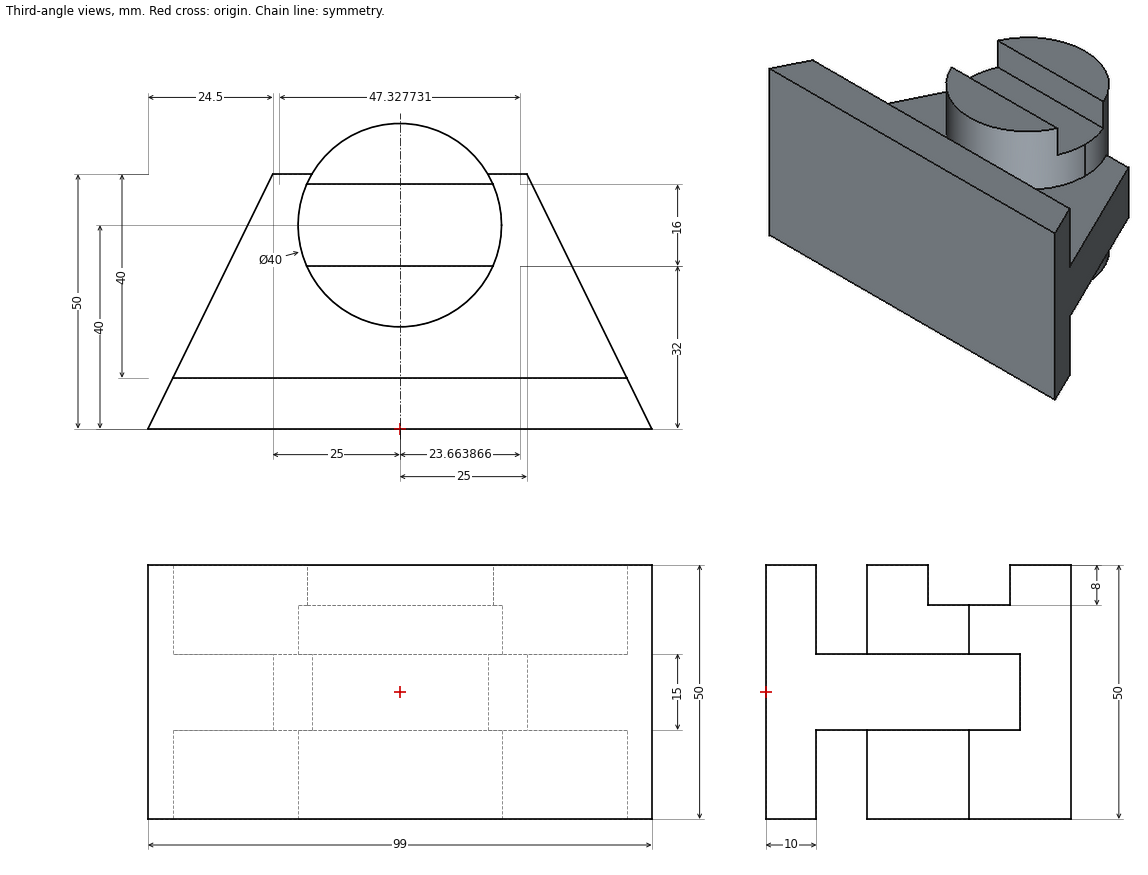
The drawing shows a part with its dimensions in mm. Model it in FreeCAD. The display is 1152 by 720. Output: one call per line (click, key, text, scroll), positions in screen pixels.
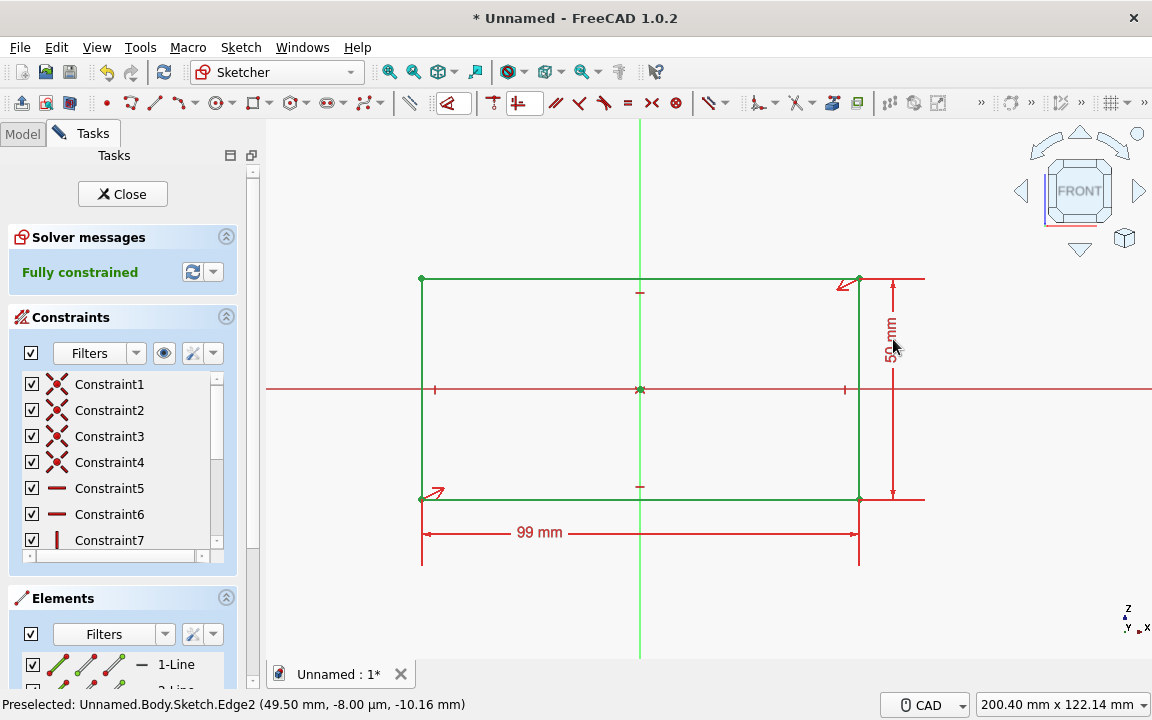
click(123, 194)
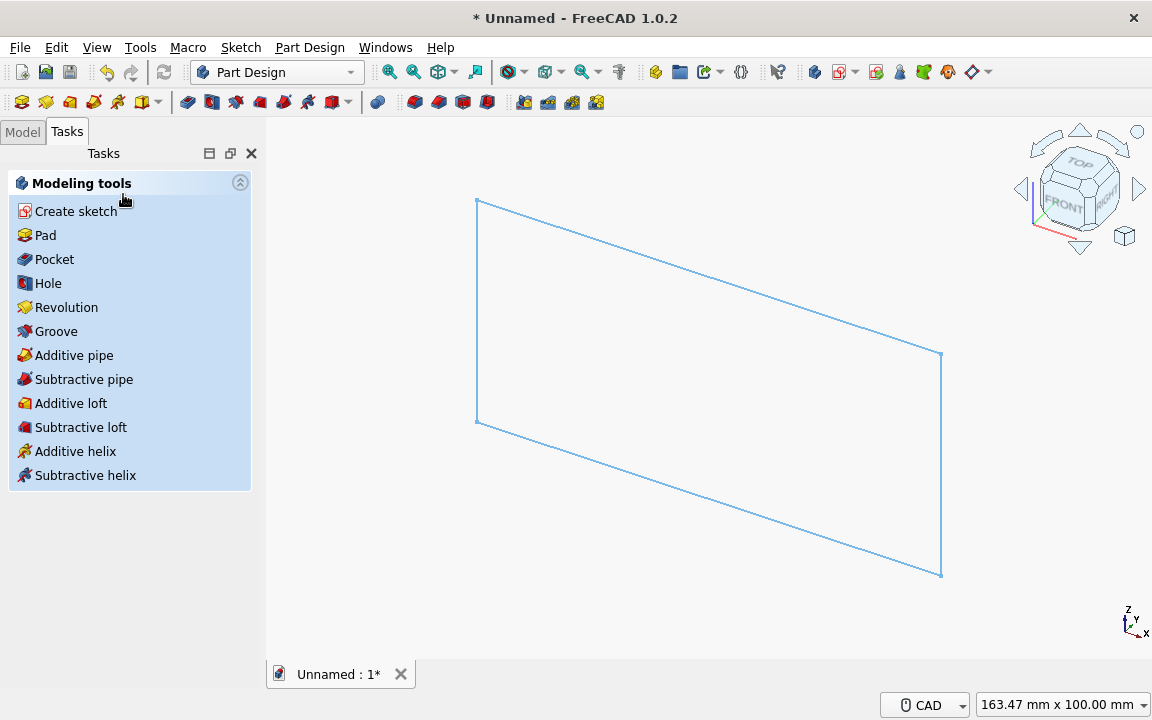
click(22, 102)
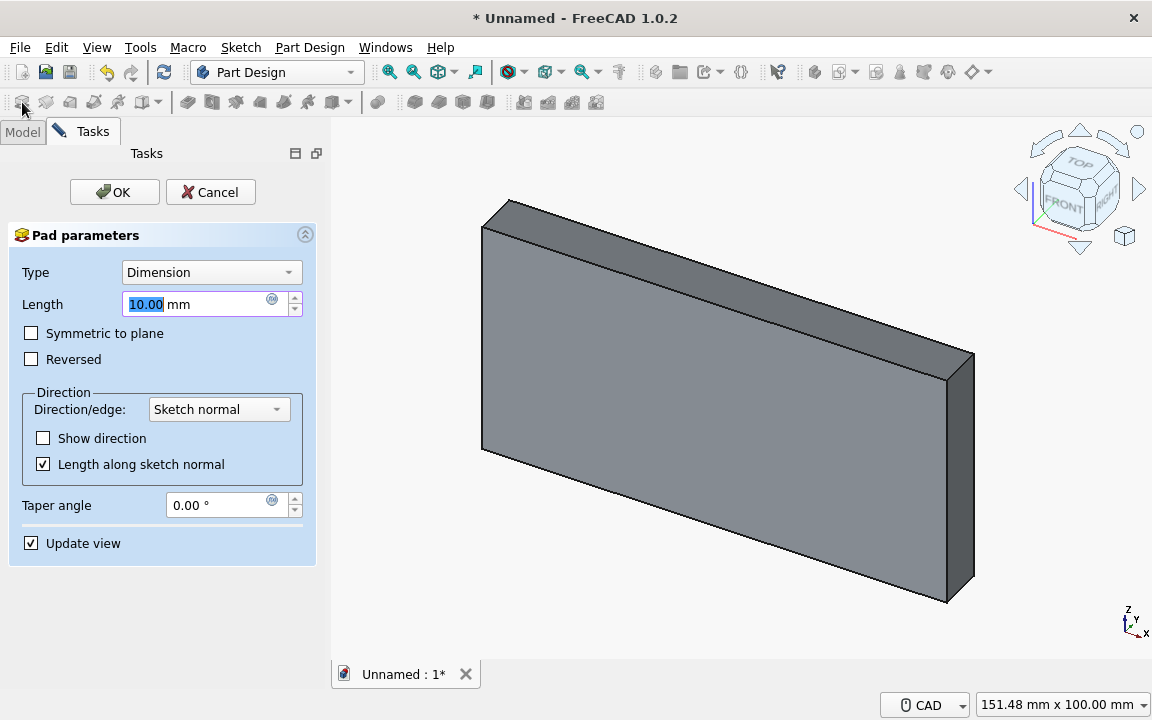
text(10)
key(Tab)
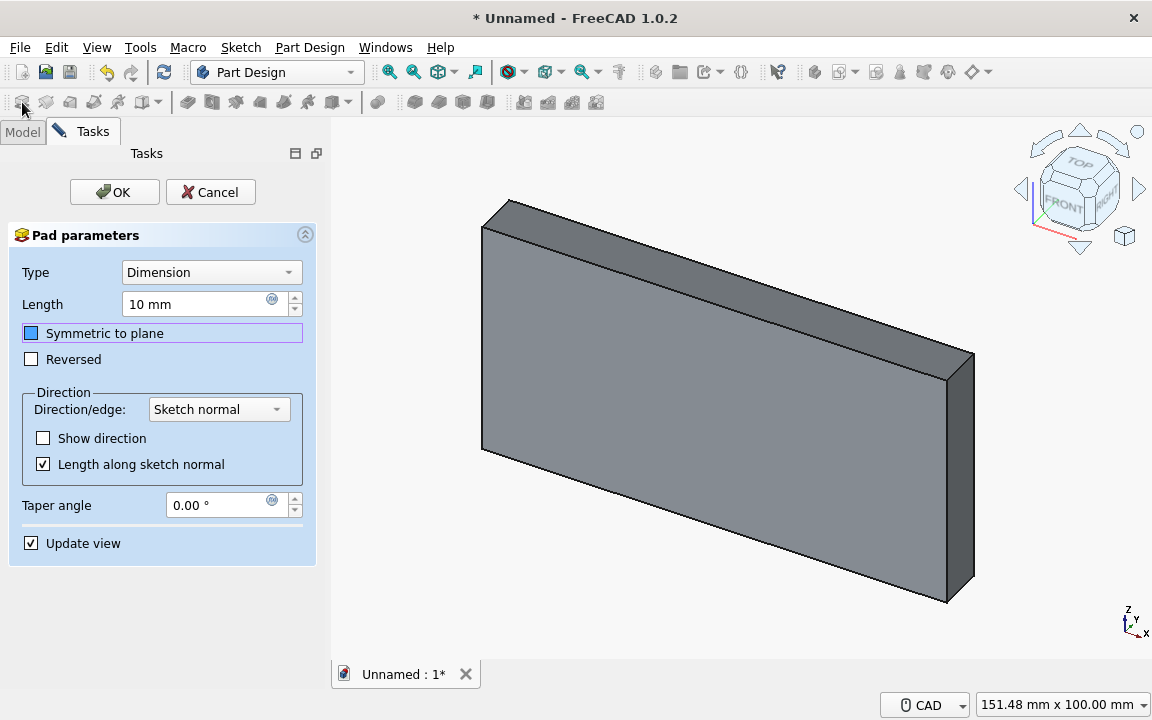
click(30, 359)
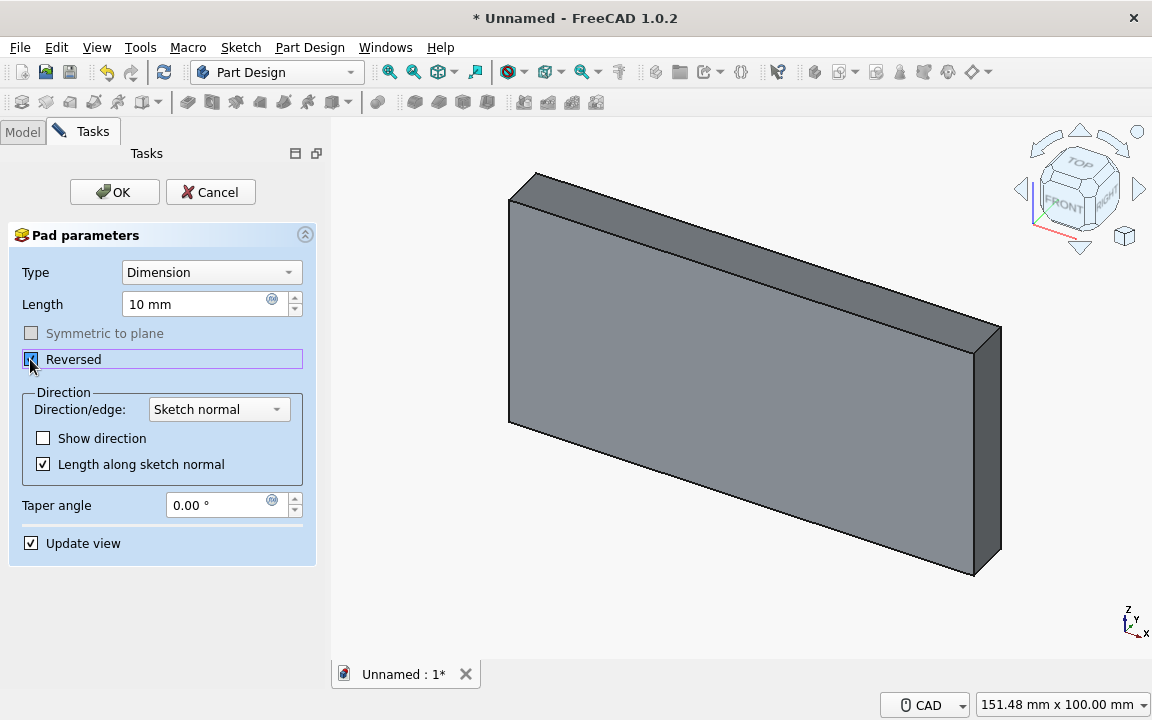
click(115, 192)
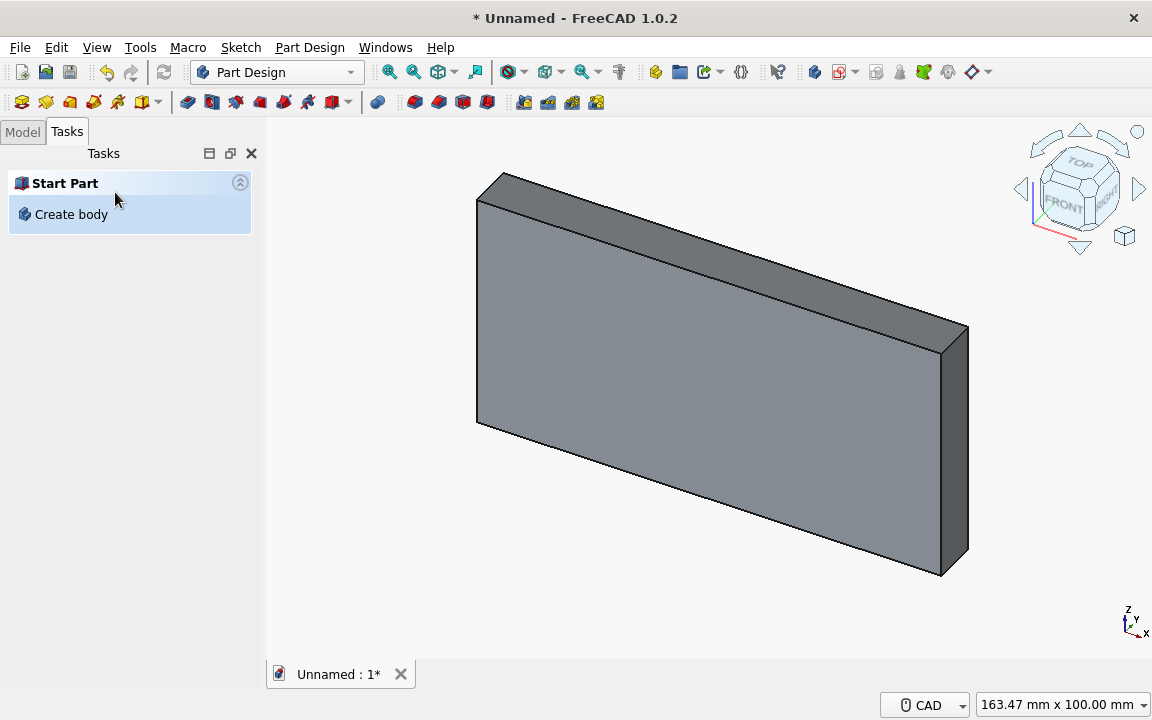
key(4)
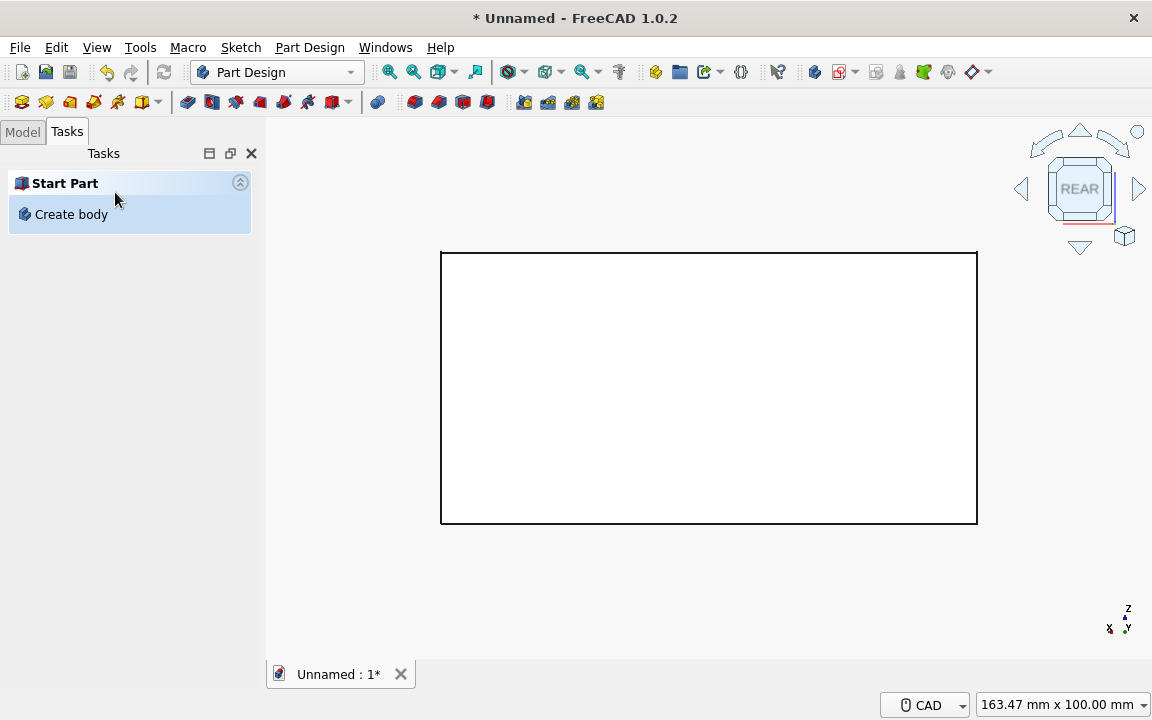
click(632, 387)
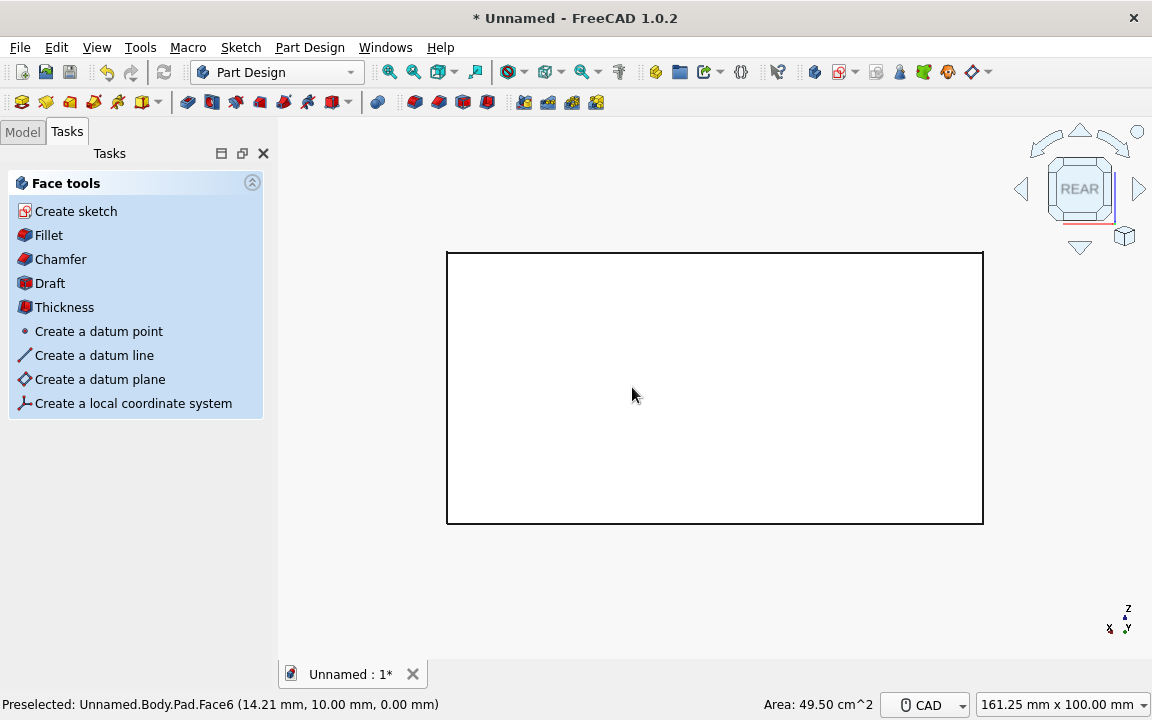
click(840, 72)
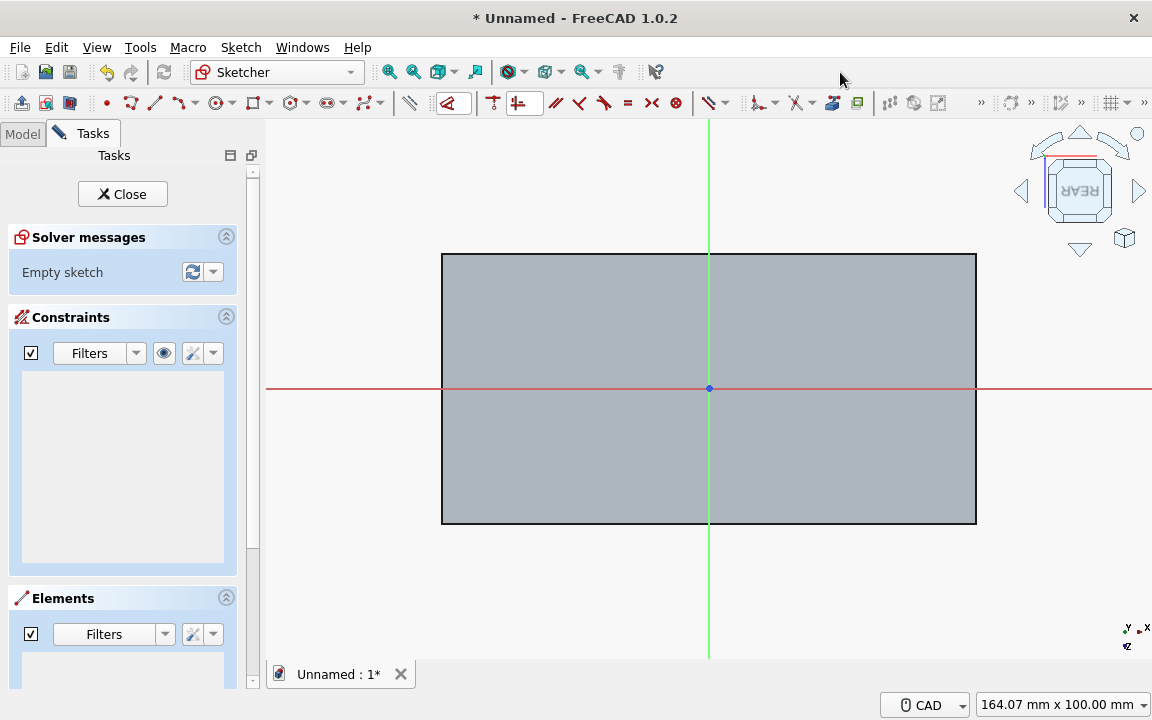
scroll(331, 389, down, 1)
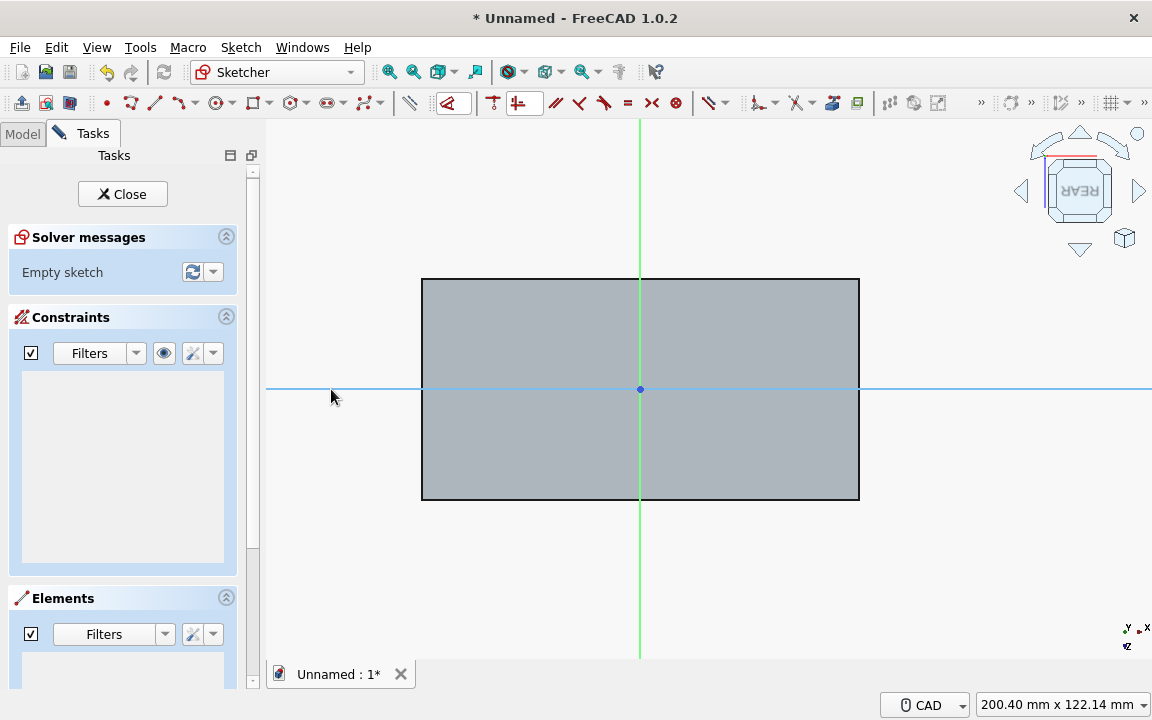
key(g)
key(v)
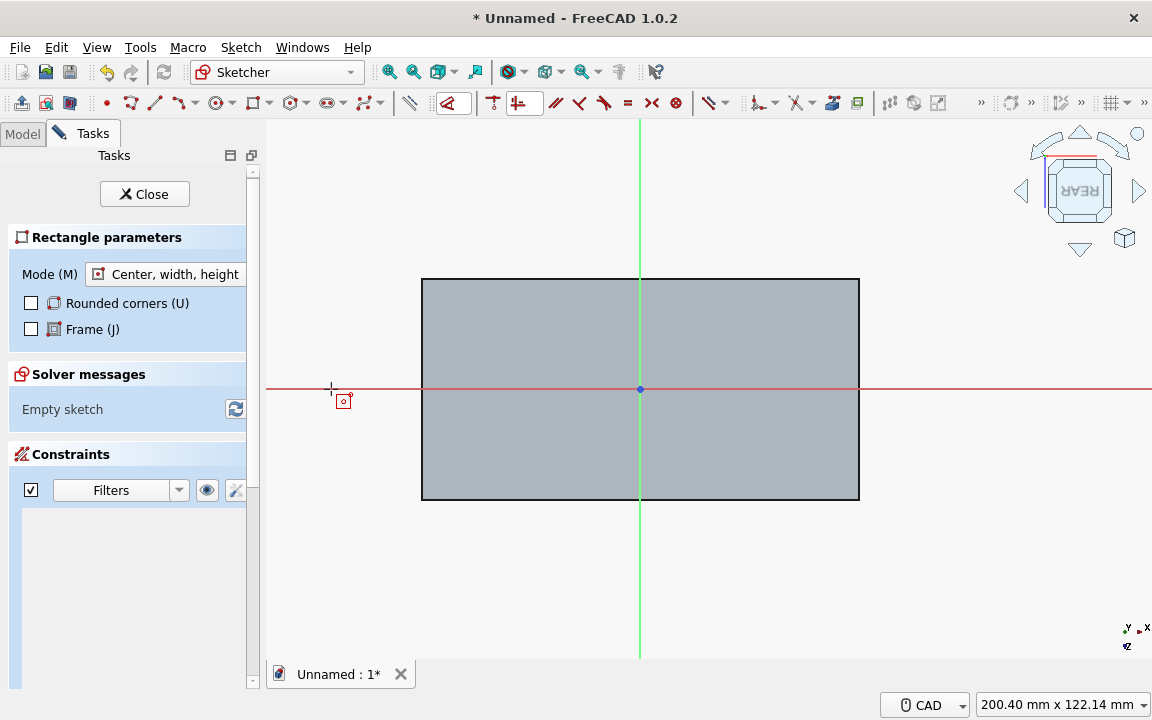
click(640, 389)
click(859, 356)
key(Escape)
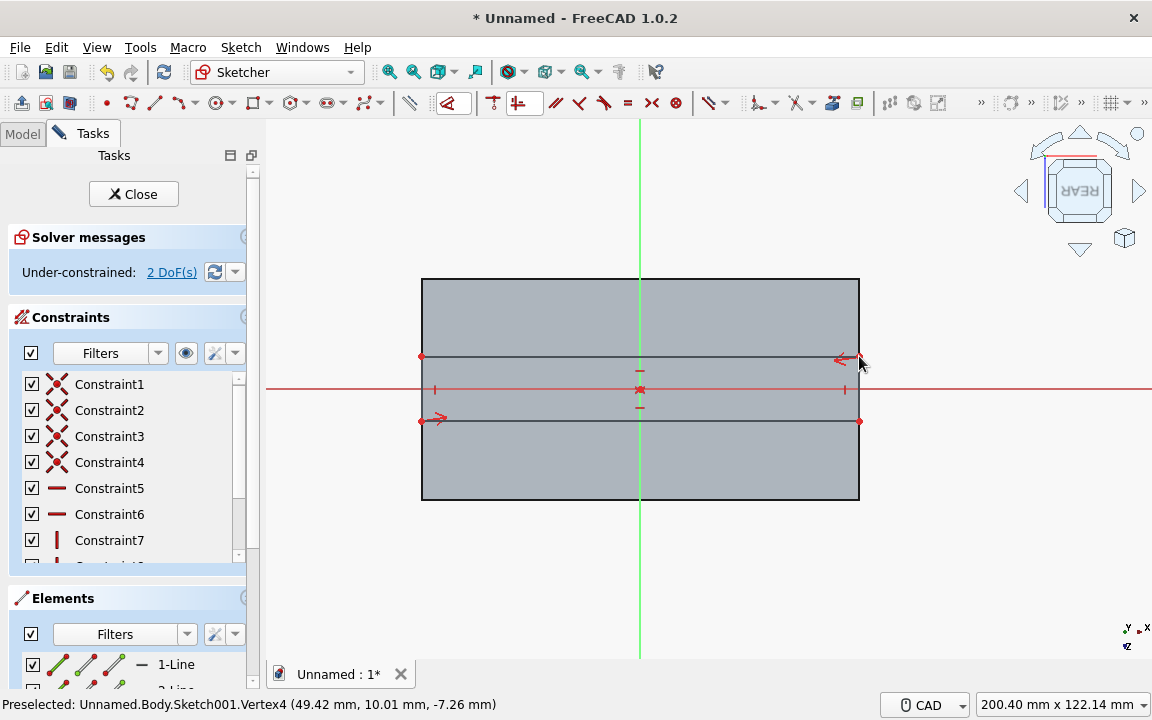
click(448, 104)